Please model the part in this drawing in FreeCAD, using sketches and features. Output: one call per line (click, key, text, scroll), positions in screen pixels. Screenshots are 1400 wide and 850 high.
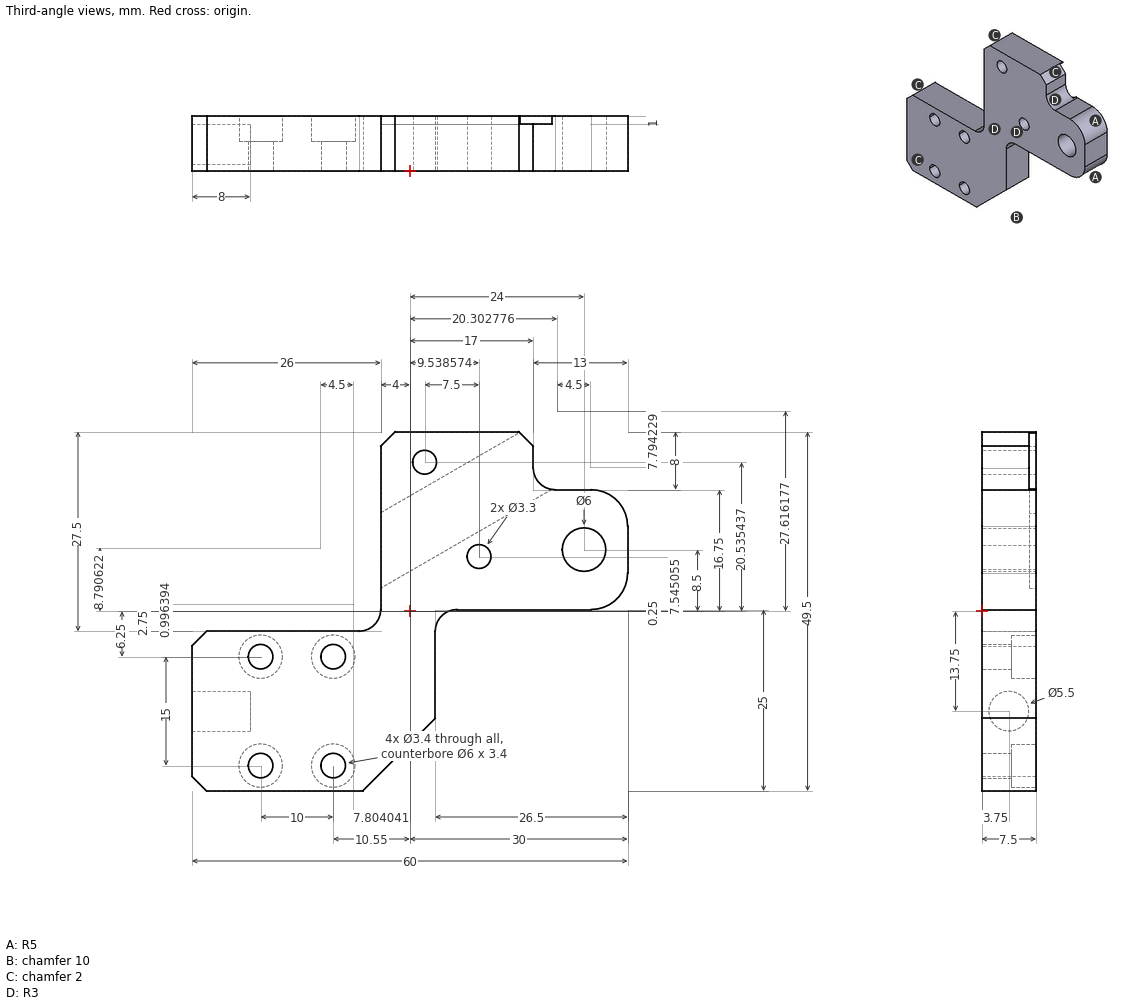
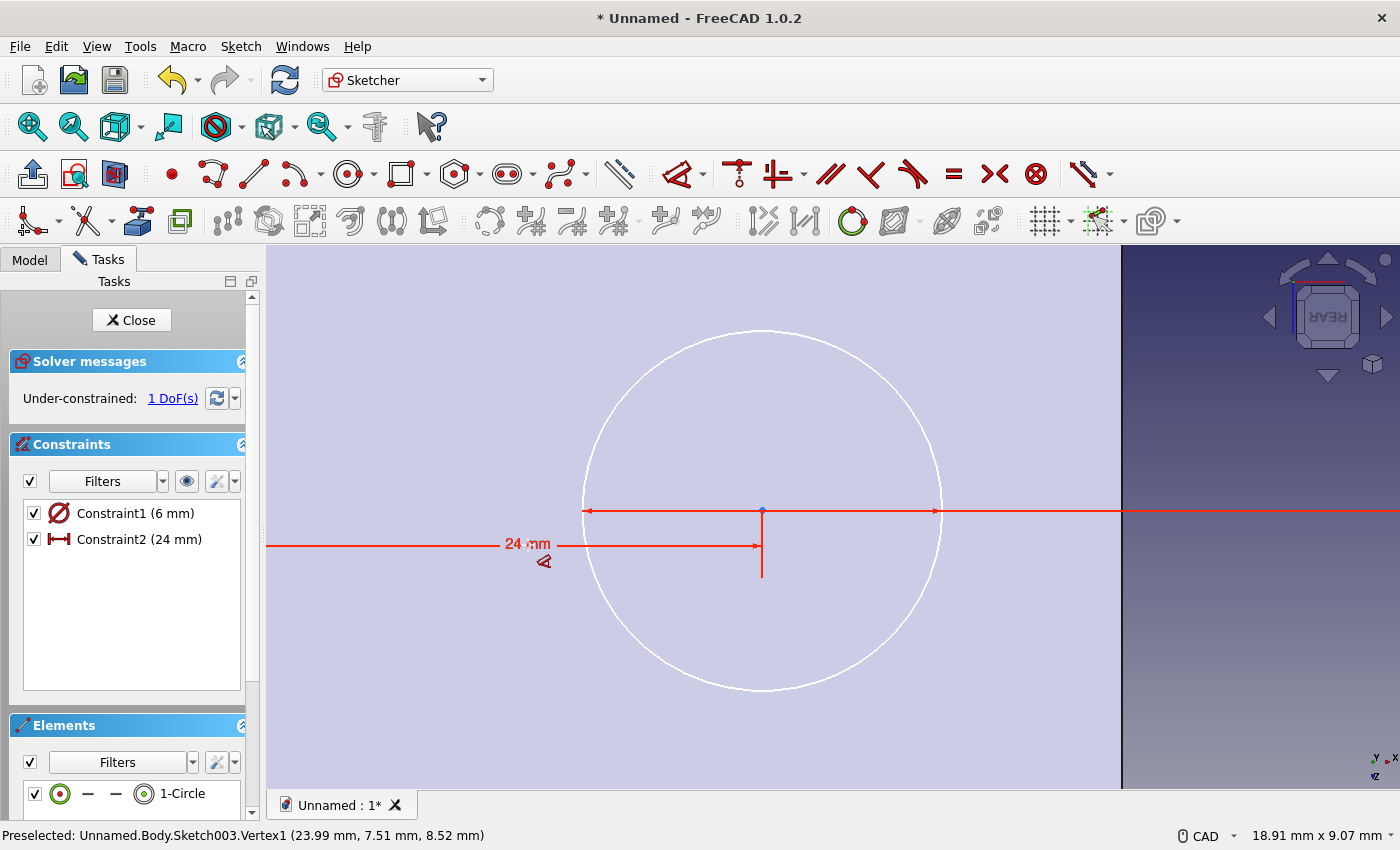
click(762, 511)
click(796, 392)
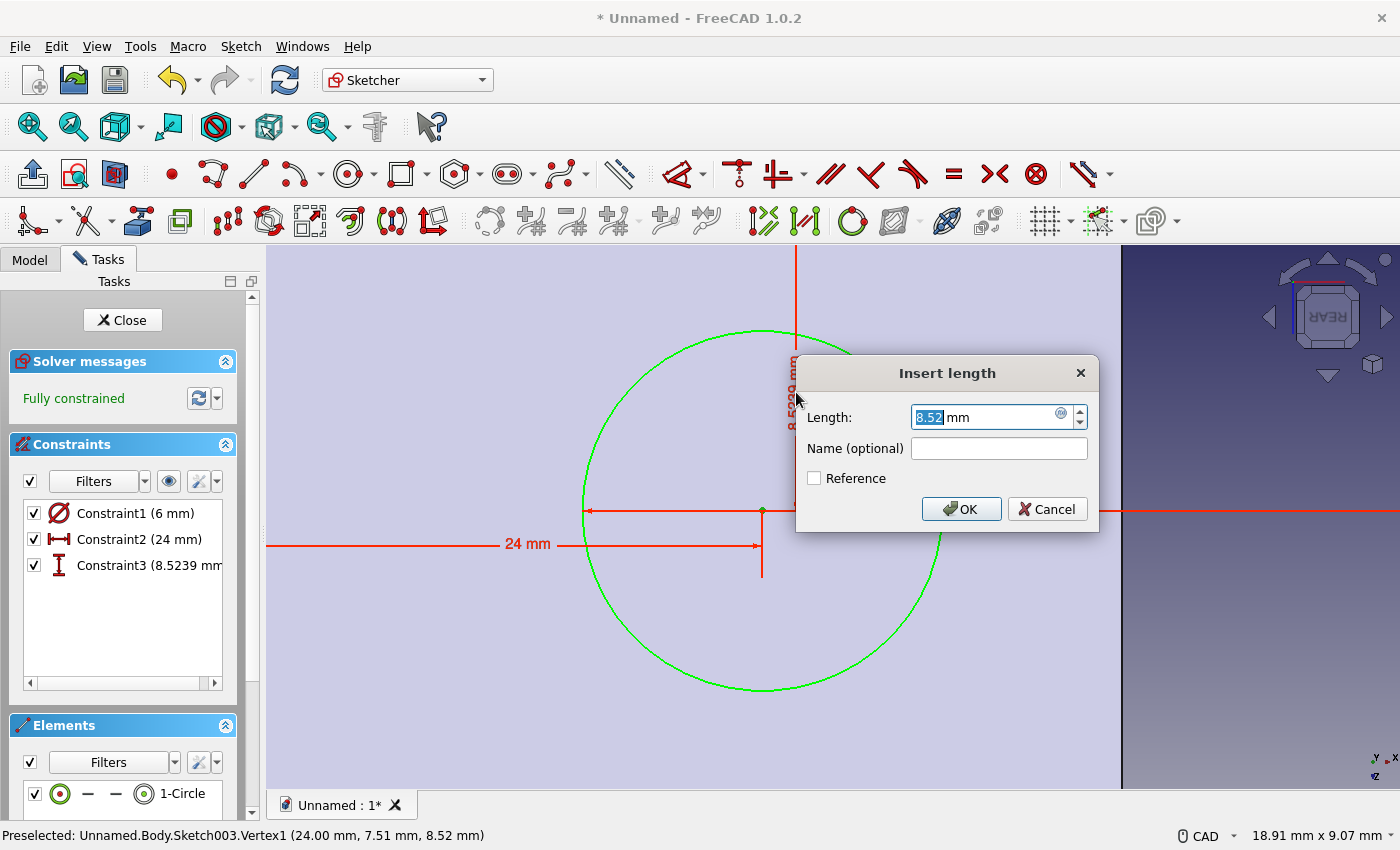
text(8.5)
key(Return)
key(Escape)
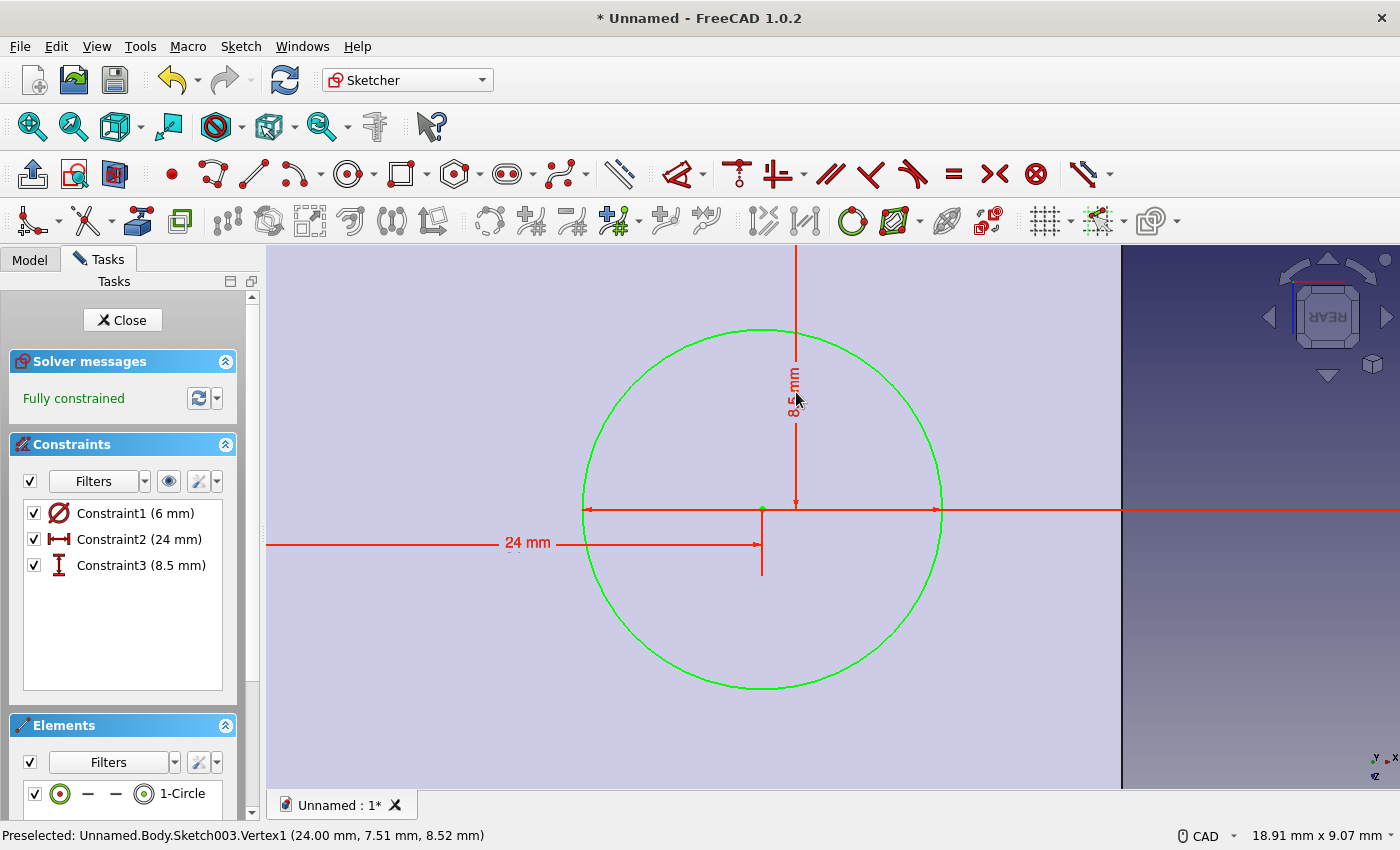
click(123, 320)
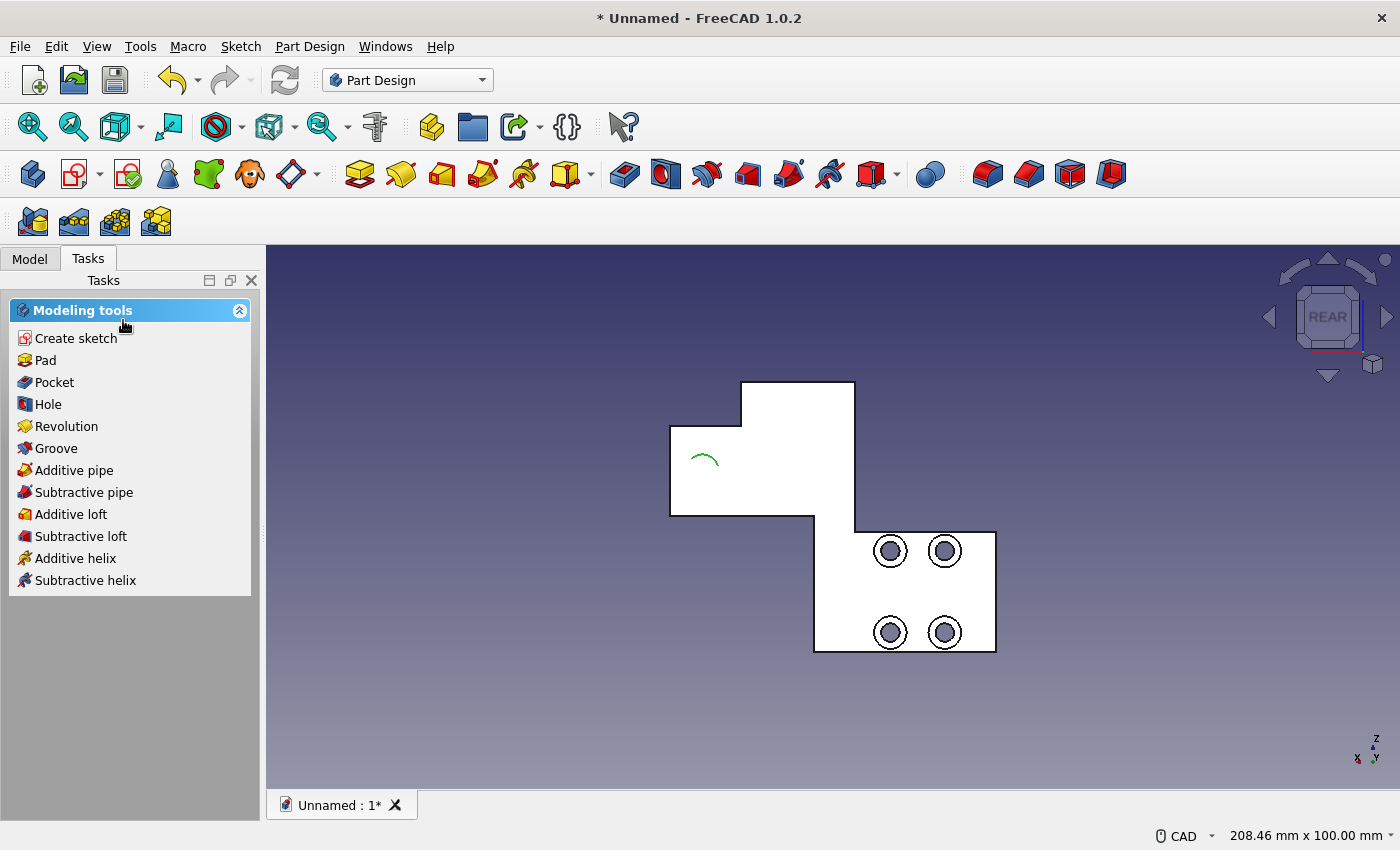
click(625, 174)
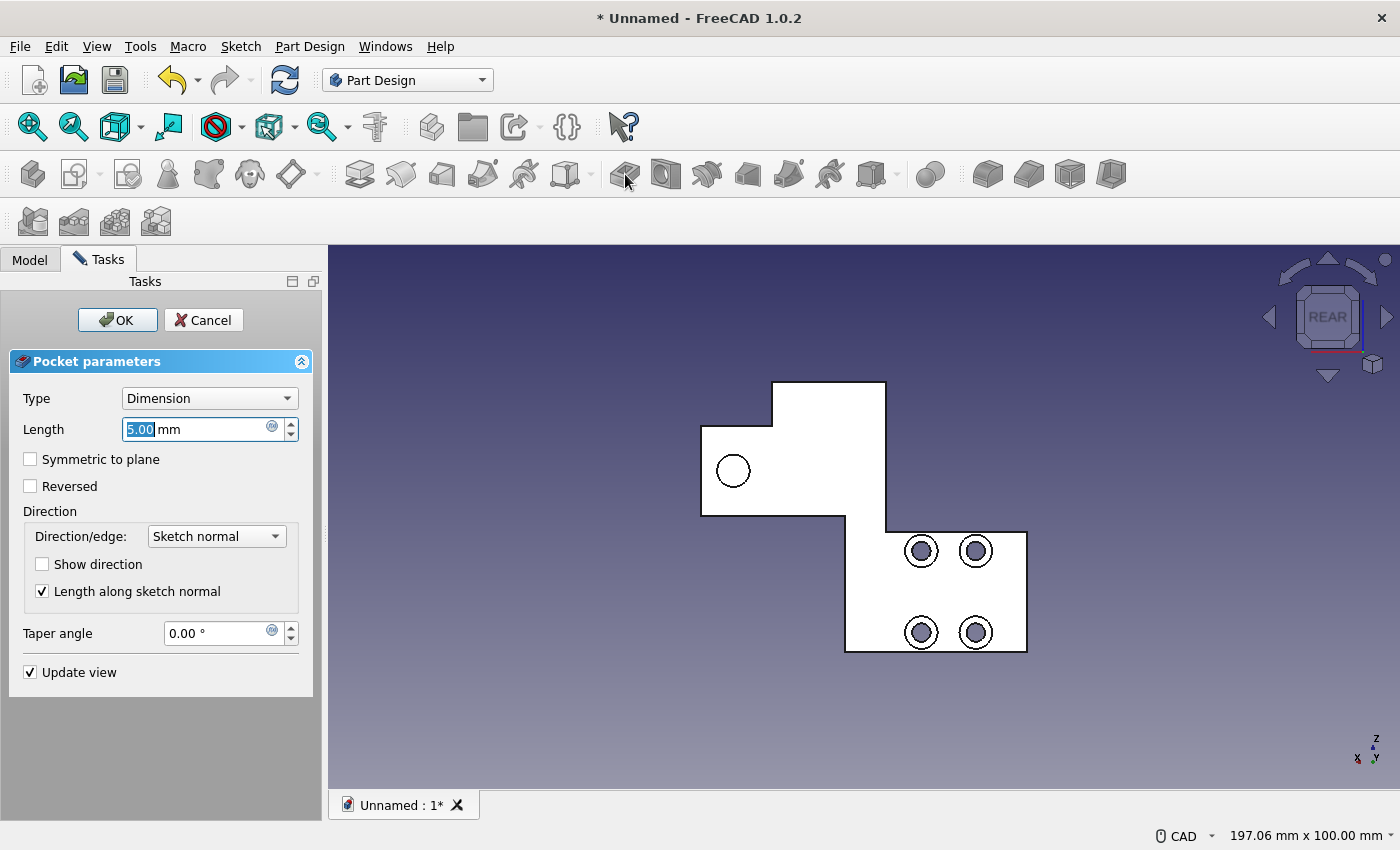
click(210, 398)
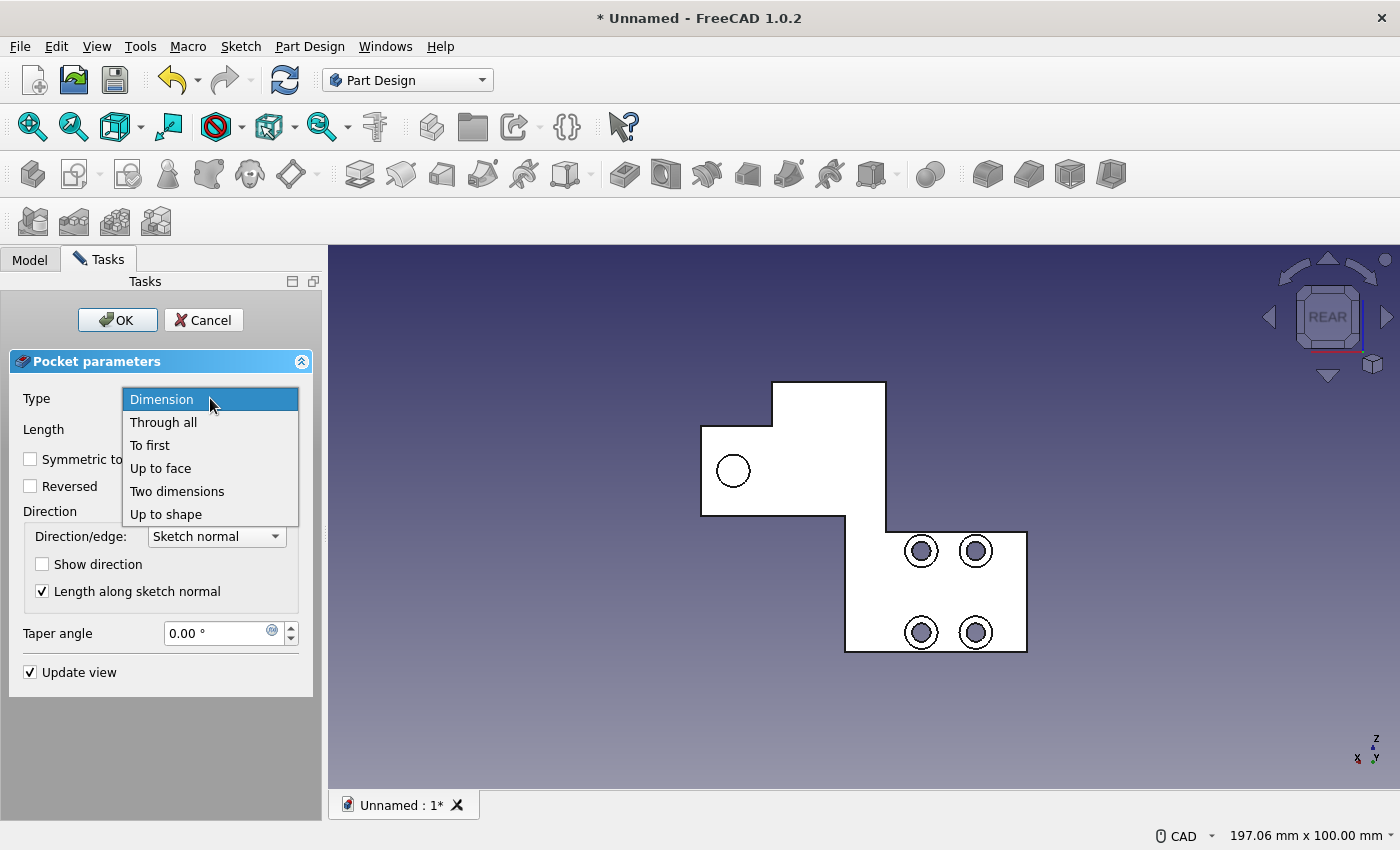
click(208, 422)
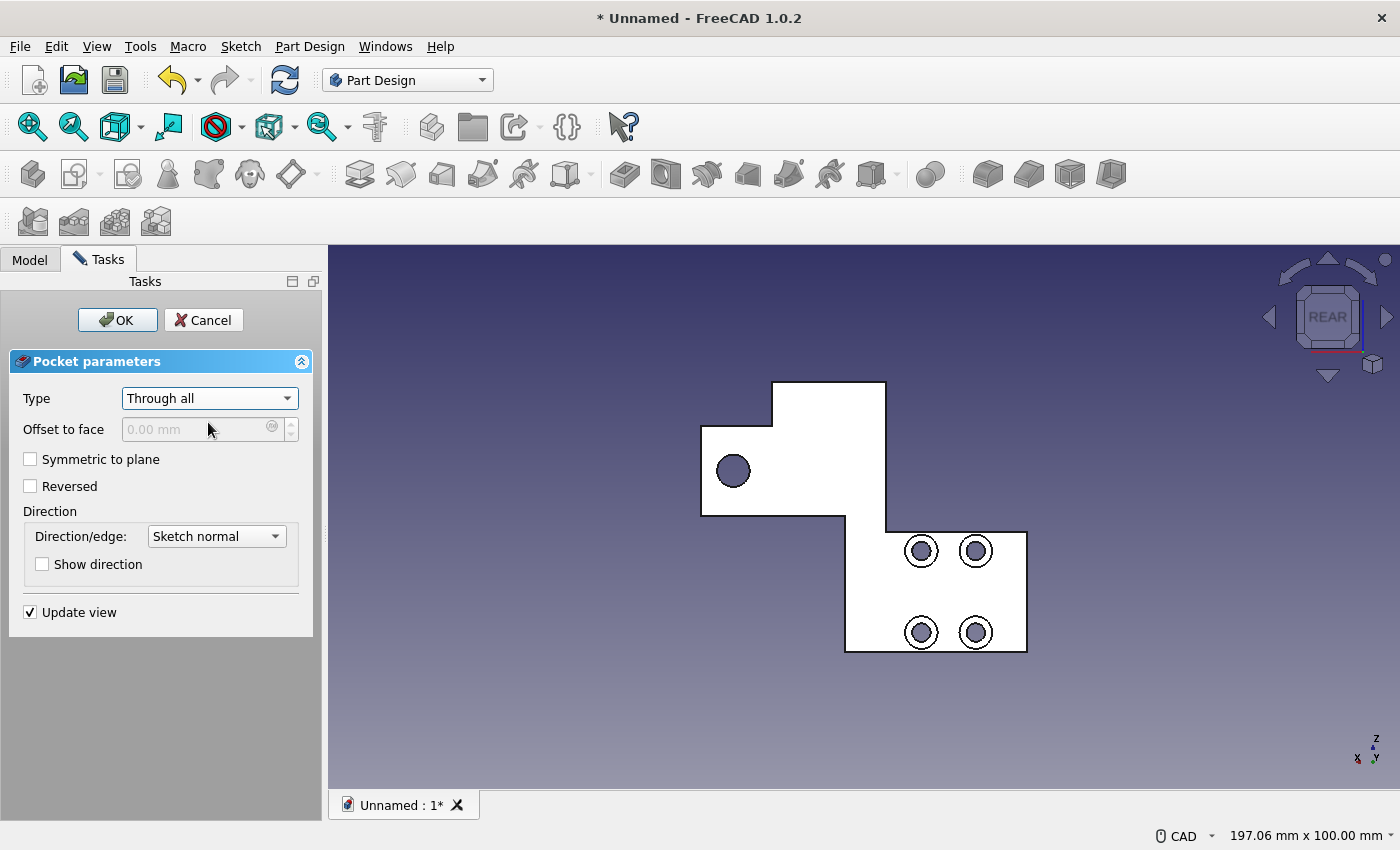
click(118, 320)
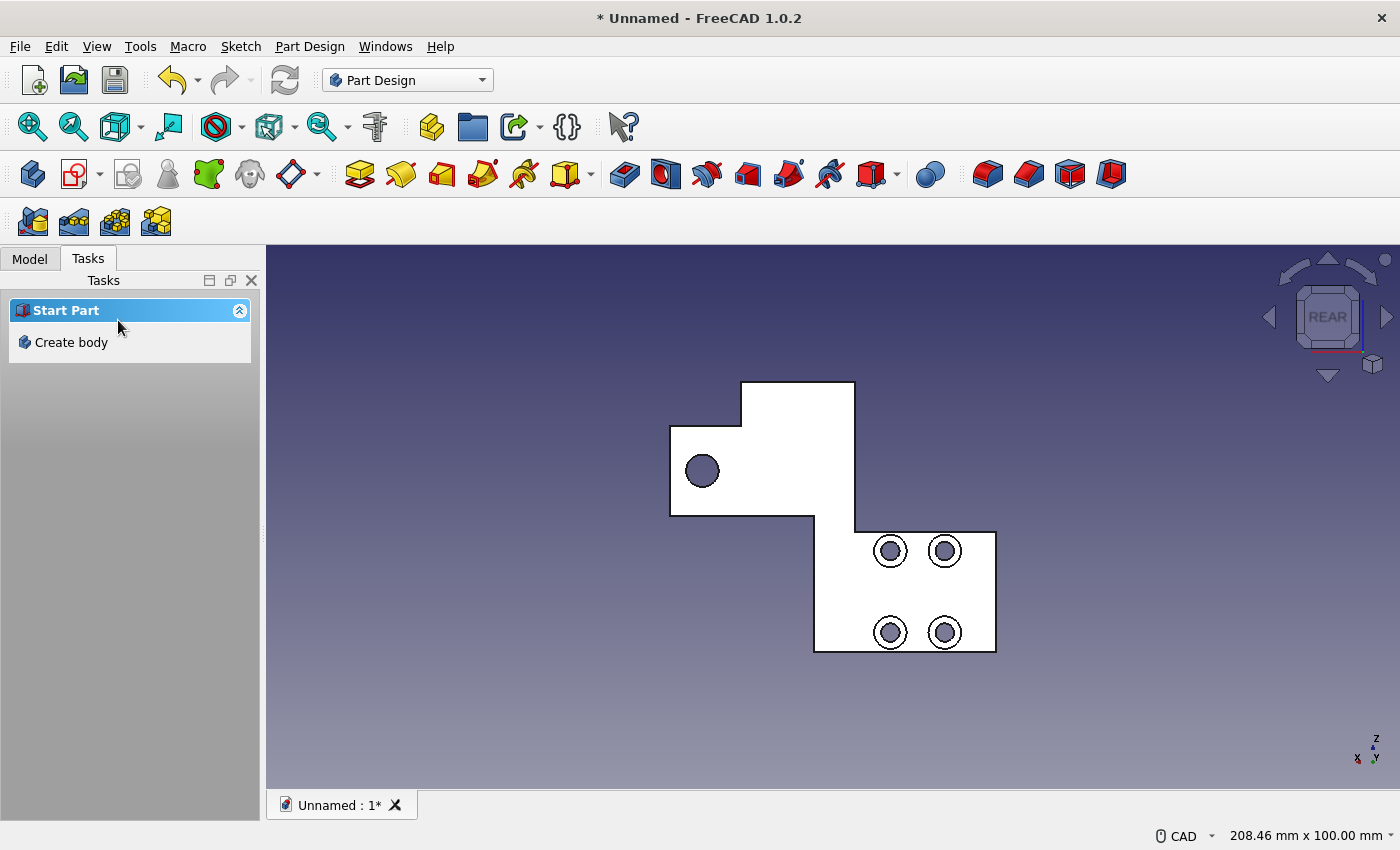
click(786, 439)